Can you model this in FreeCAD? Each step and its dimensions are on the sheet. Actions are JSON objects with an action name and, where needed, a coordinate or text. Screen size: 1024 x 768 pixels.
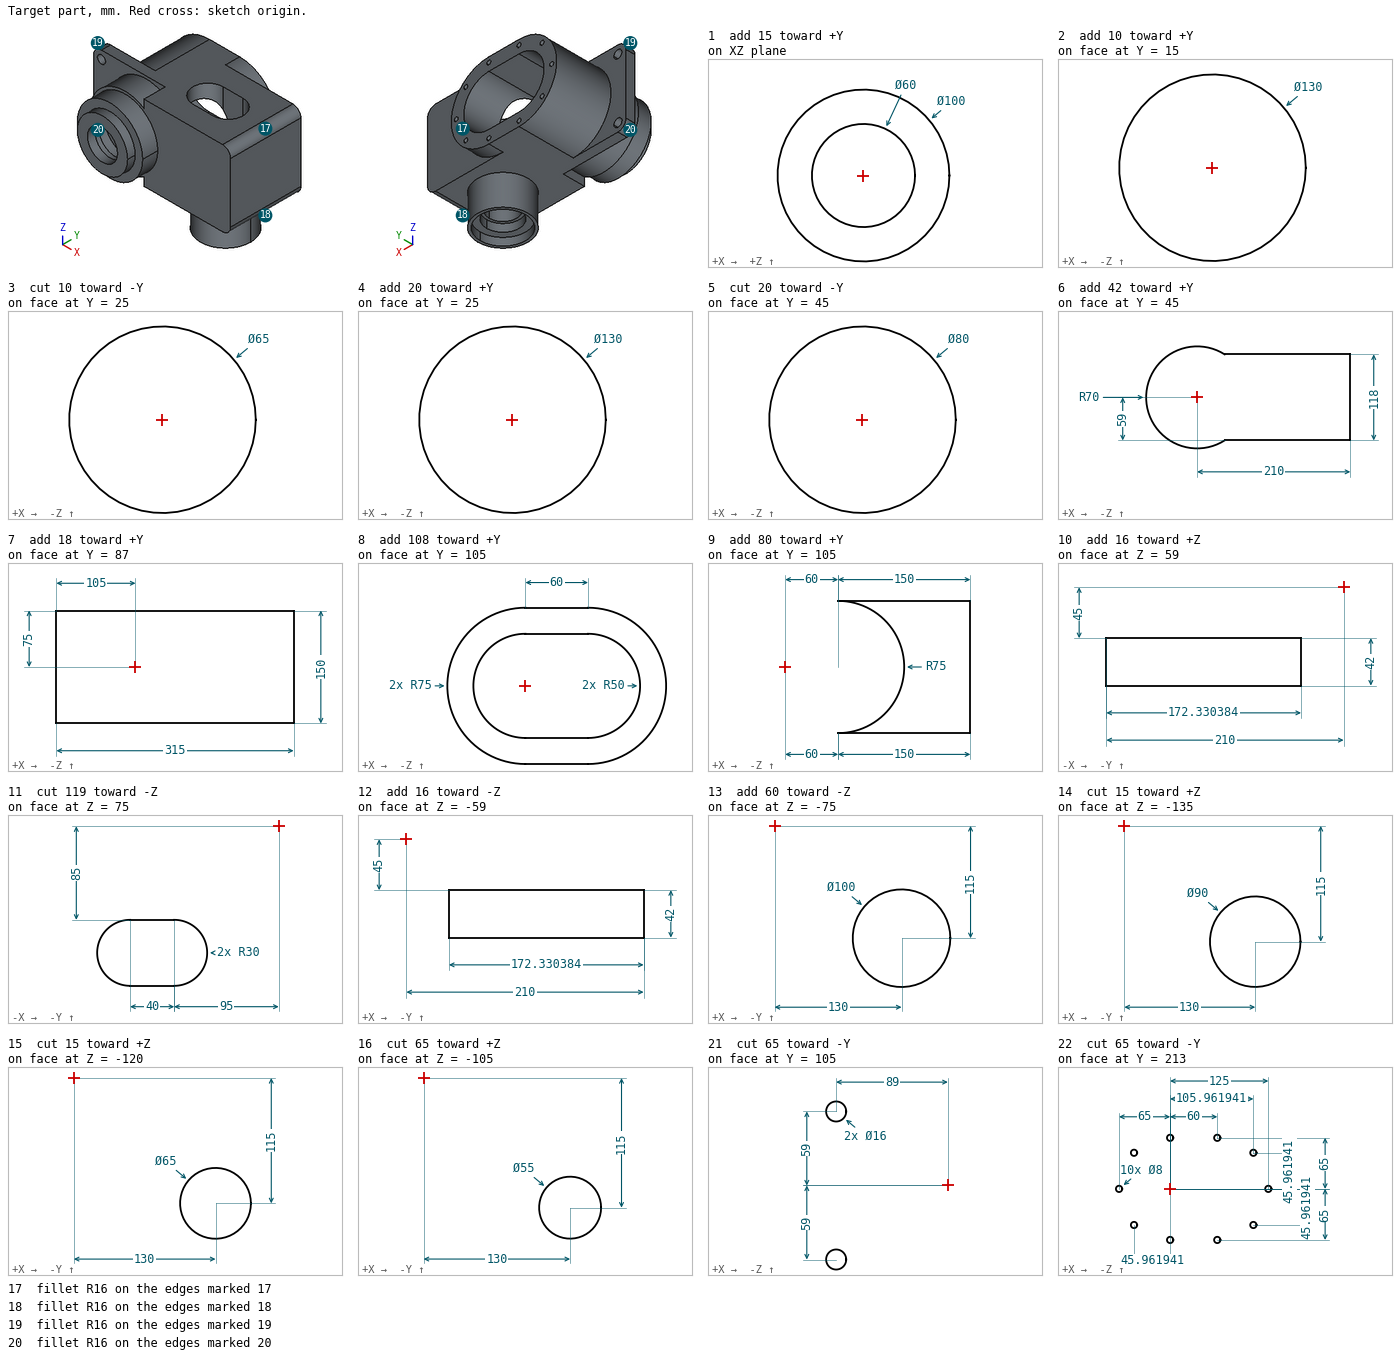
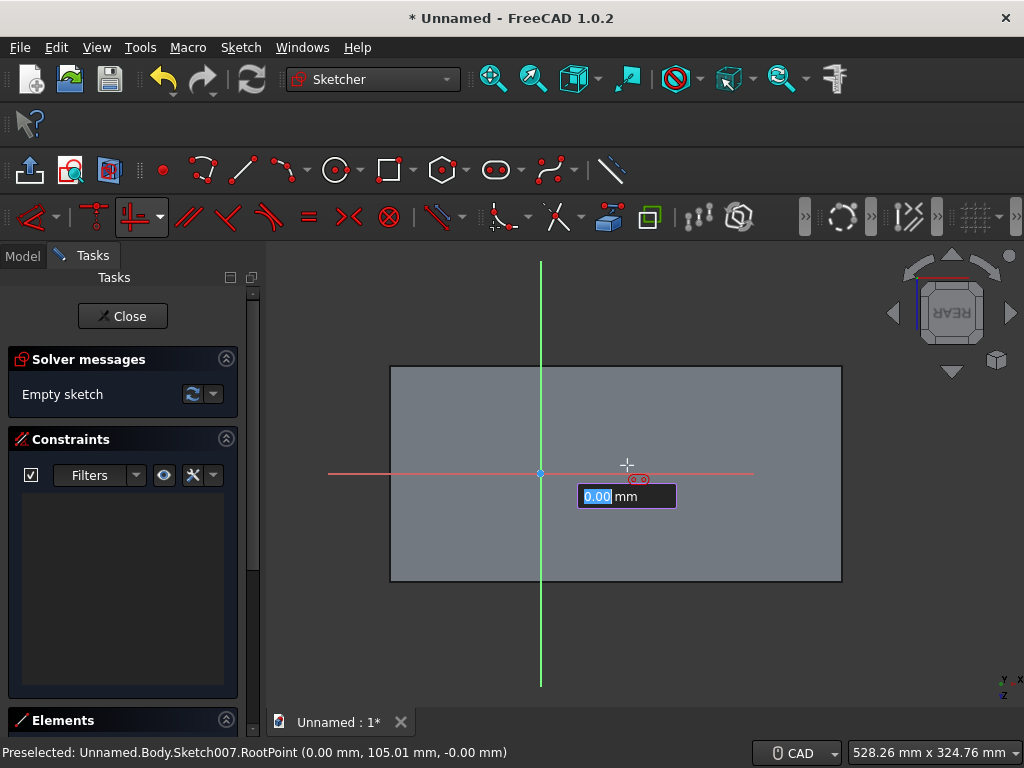
{"action": "left_click", "coordinate": [584, 366]}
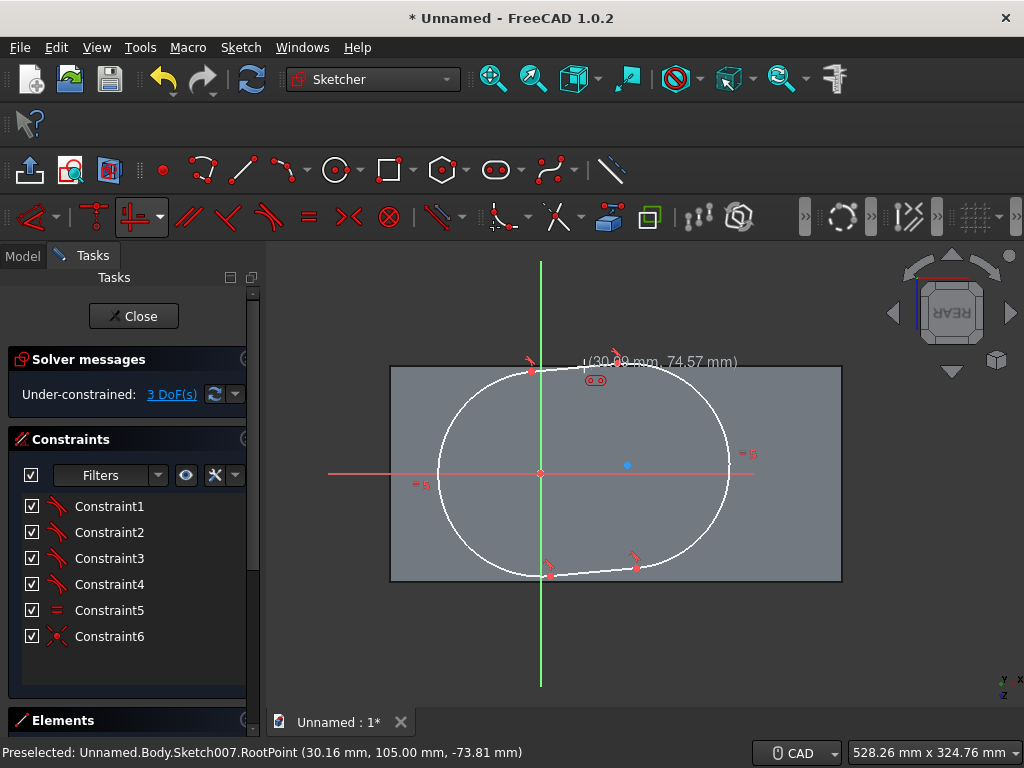
{"action": "left_click", "coordinate": [541, 474]}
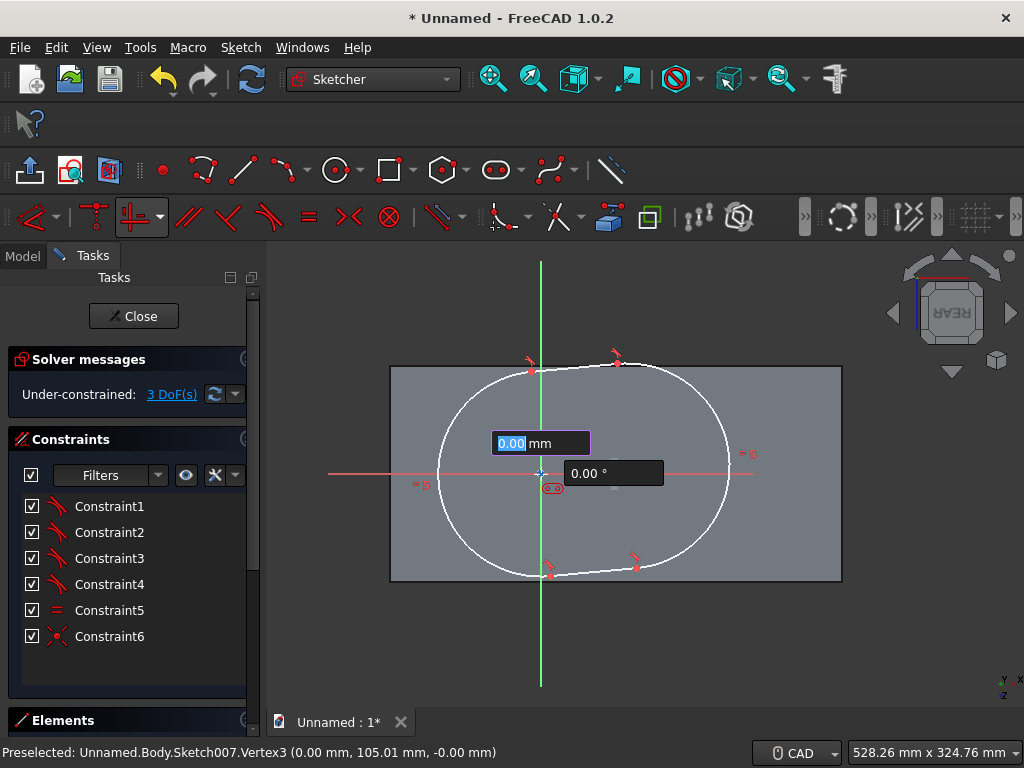
{"action": "left_click", "coordinate": [627, 466]}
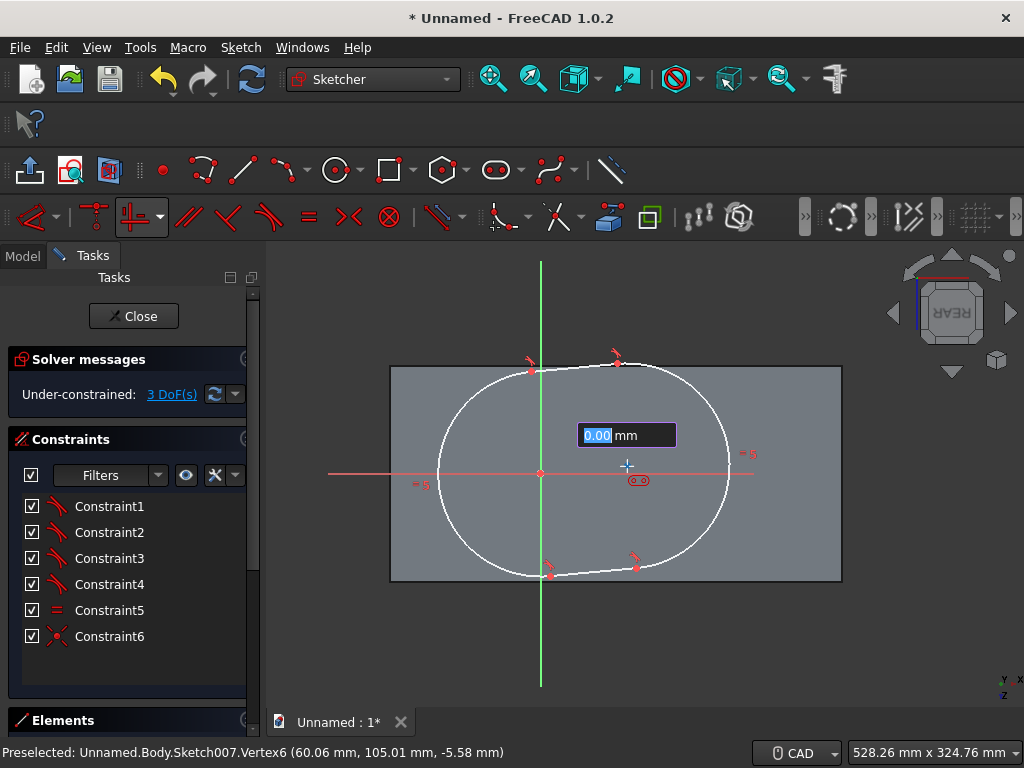
{"action": "left_click", "coordinate": [584, 402]}
{"action": "key", "text": "Escape"}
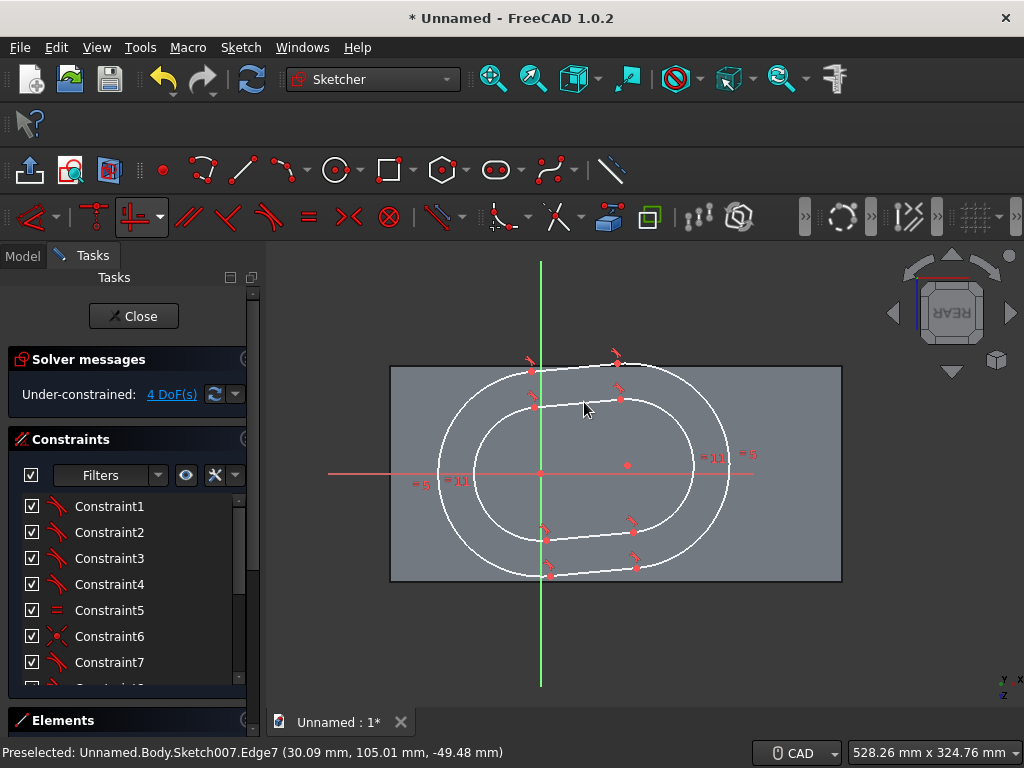
{"action": "left_click", "coordinate": [557, 369]}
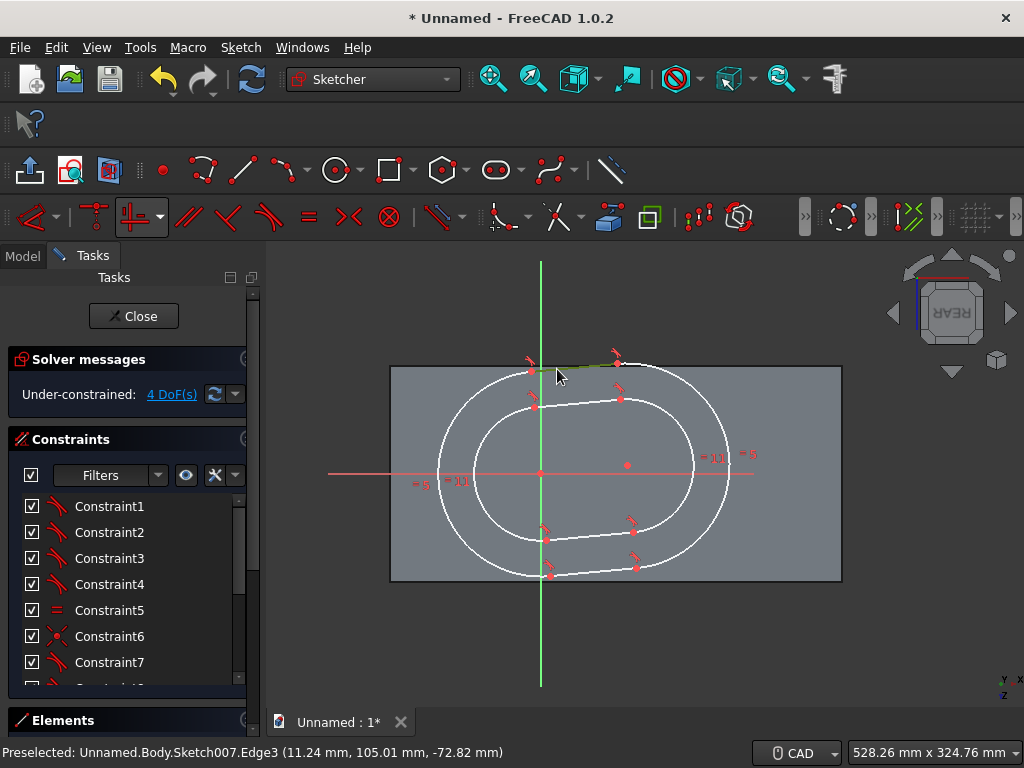
{"action": "key", "text": "h"}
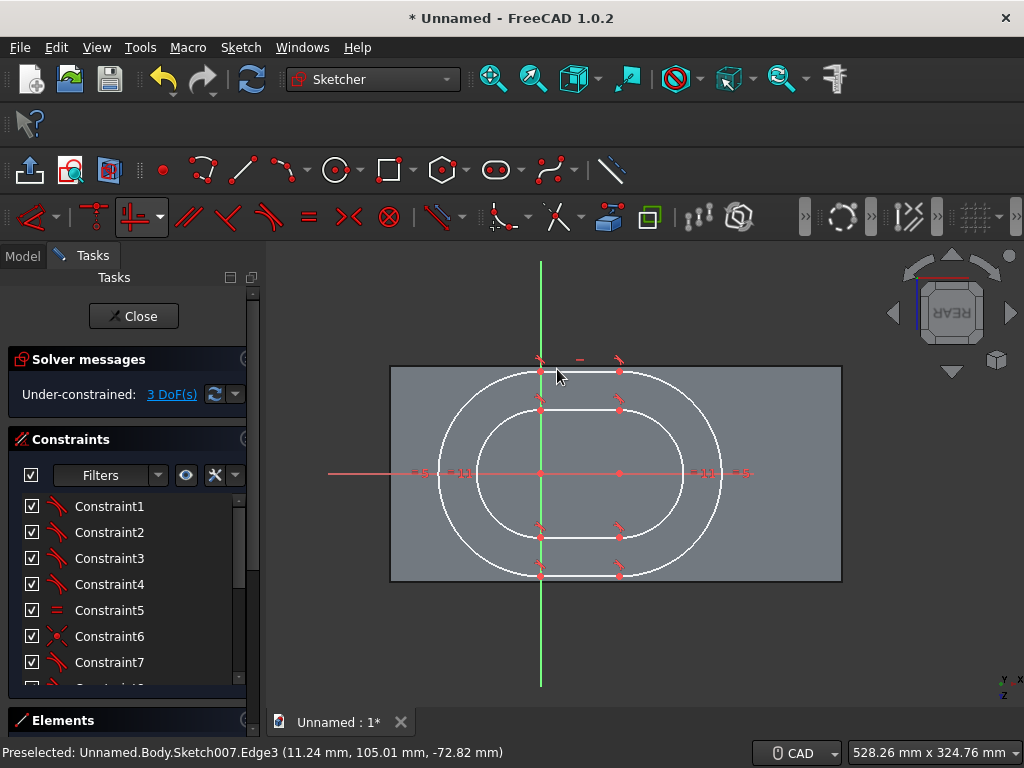
{"action": "left_click", "coordinate": [32, 218]}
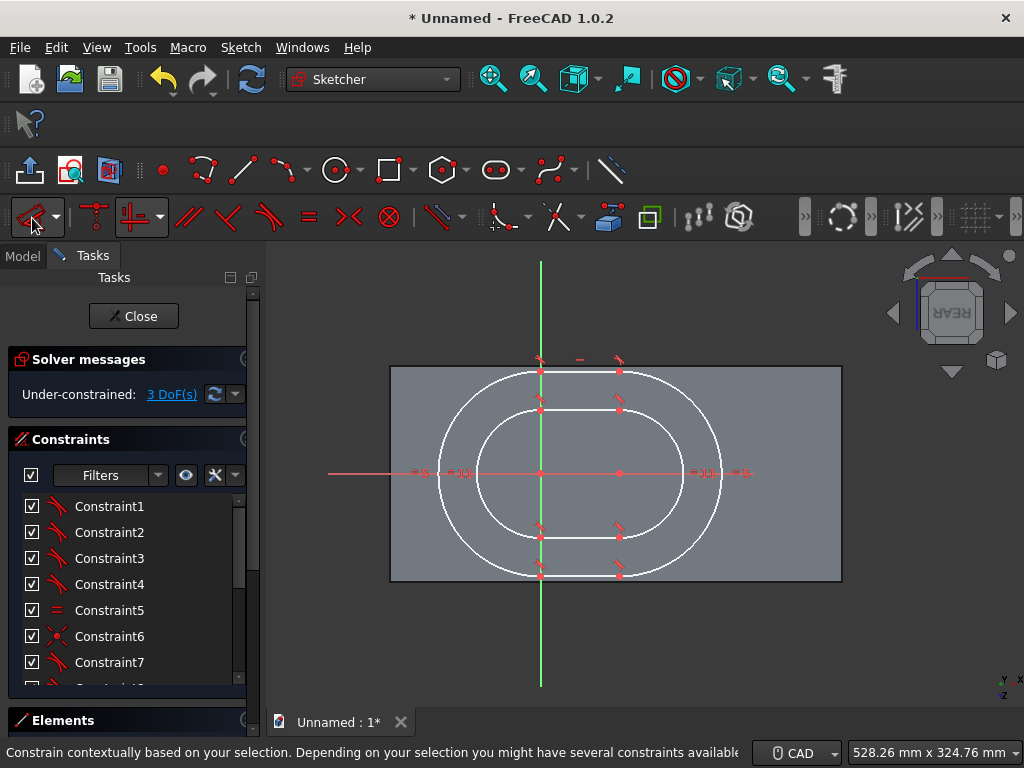
{"action": "left_click", "coordinate": [458, 414]}
{"action": "left_click", "coordinate": [432, 395]}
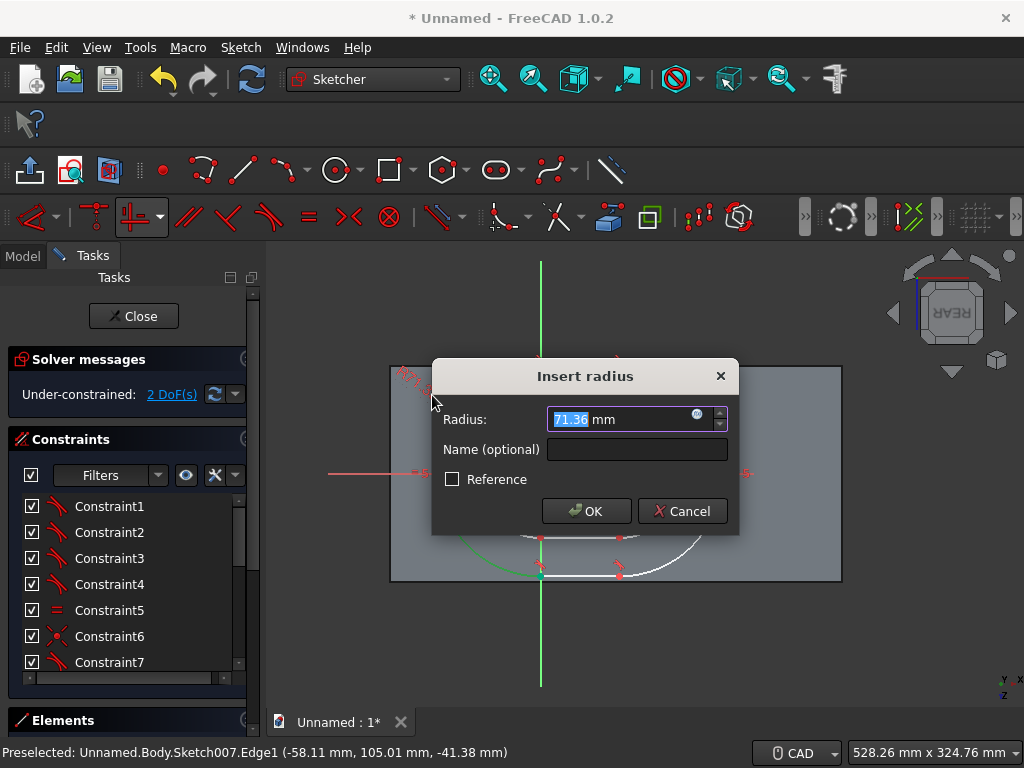
{"action": "type", "text": "75"}
{"action": "key", "text": "Return"}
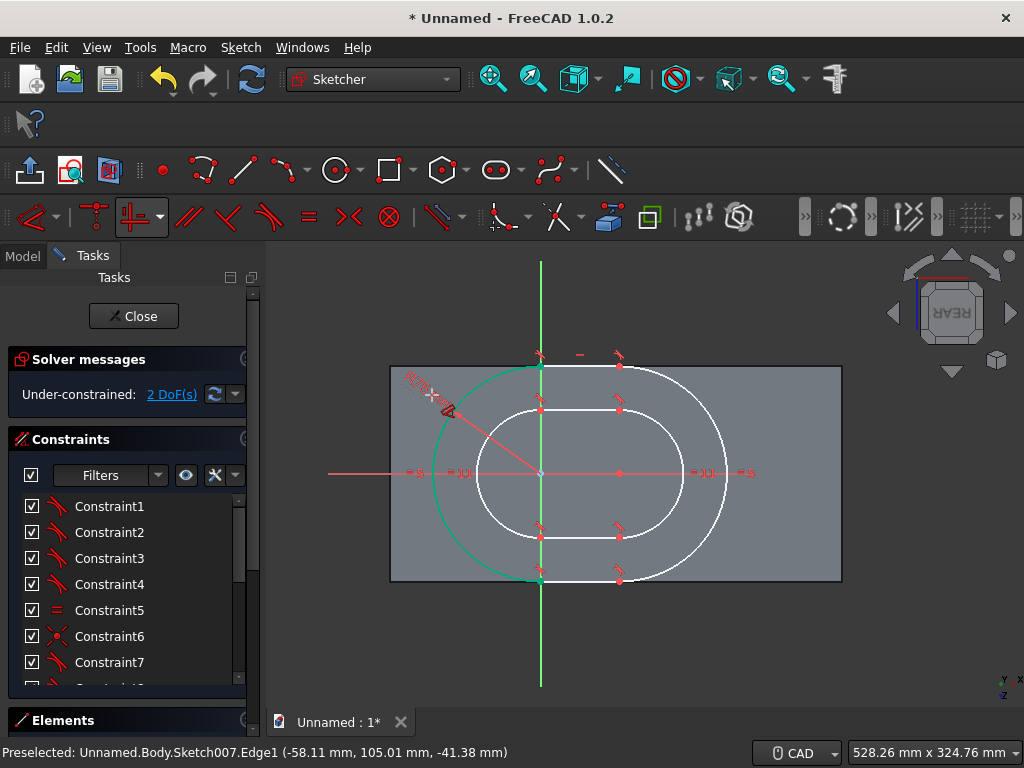
{"action": "left_click", "coordinate": [489, 436]}
{"action": "left_click", "coordinate": [598, 396]}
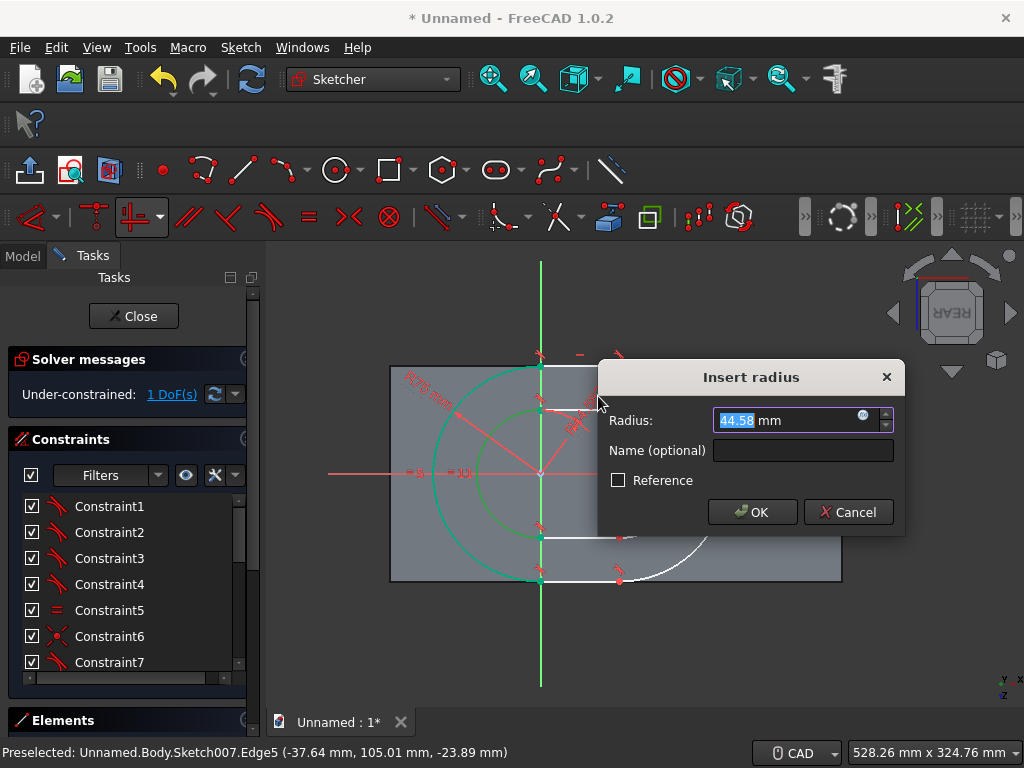
{"action": "type", "text": "50"}
{"action": "key", "text": "Return"}